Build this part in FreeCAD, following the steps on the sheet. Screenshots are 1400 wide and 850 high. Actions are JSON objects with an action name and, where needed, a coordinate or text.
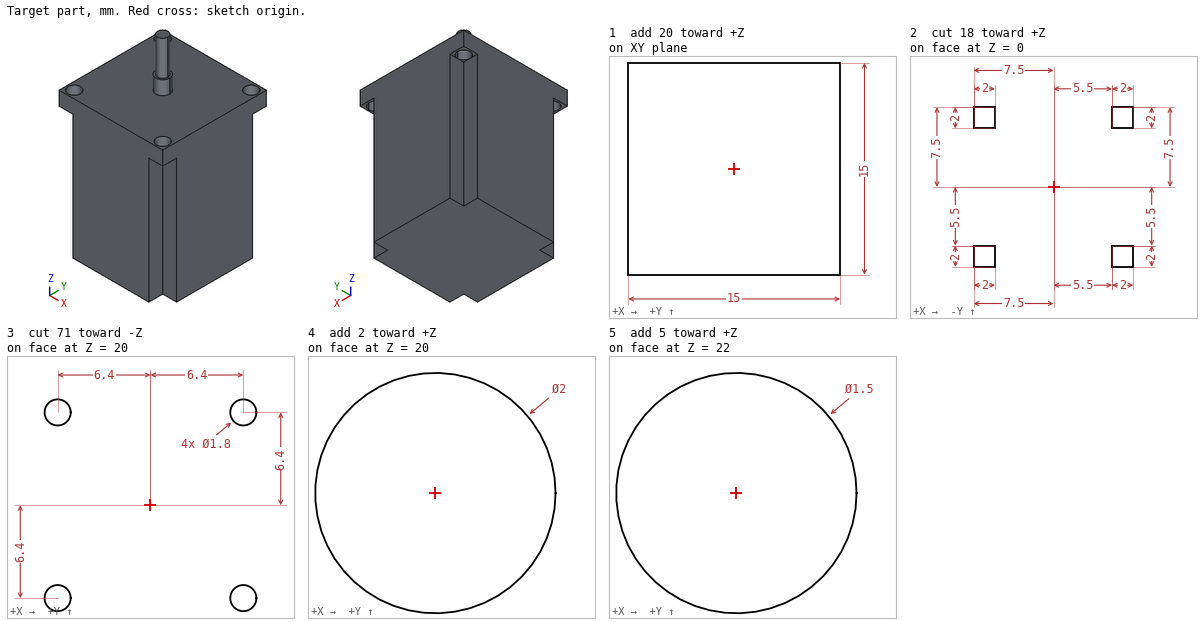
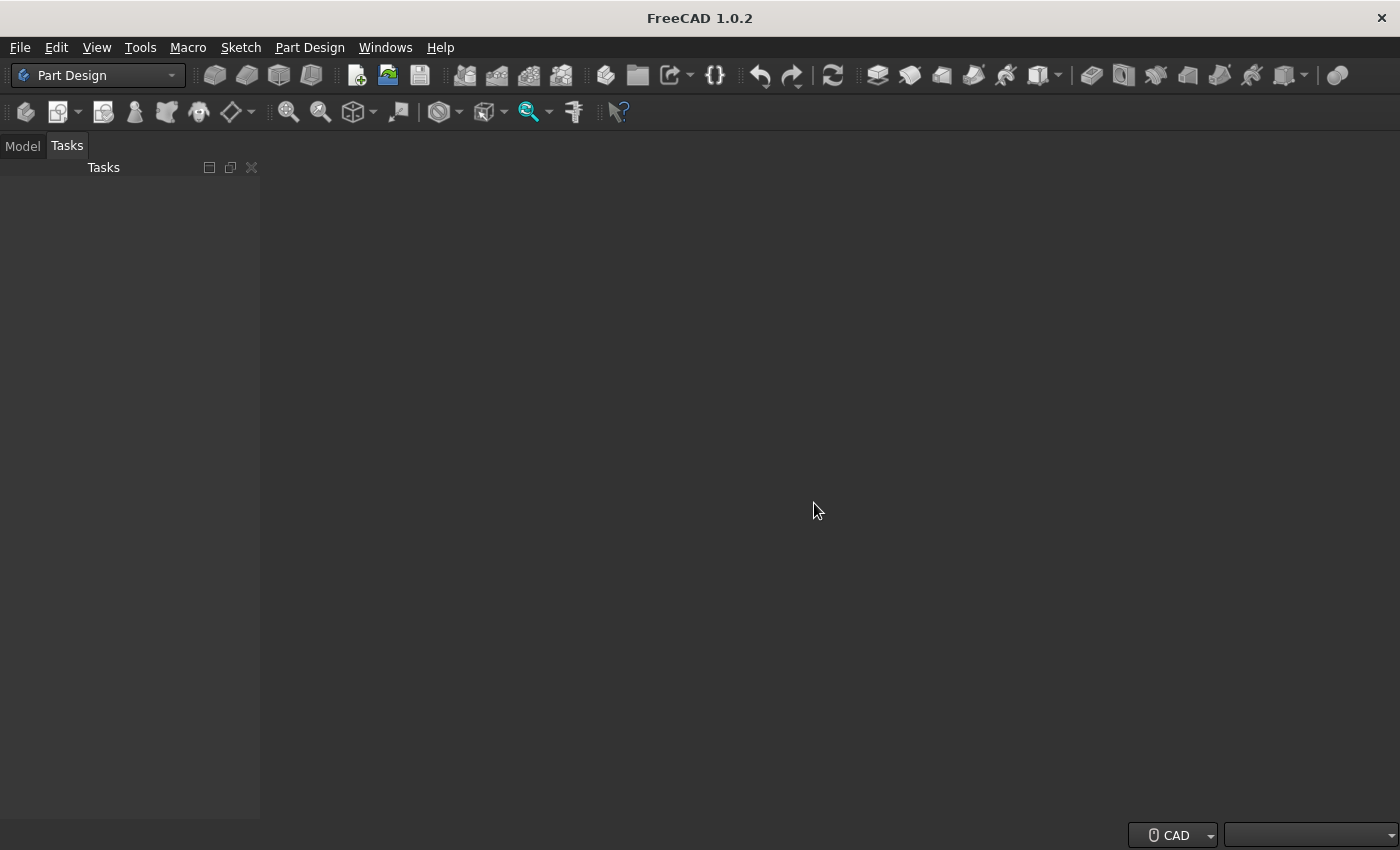
{"action": "left_click", "coordinate": [356, 76]}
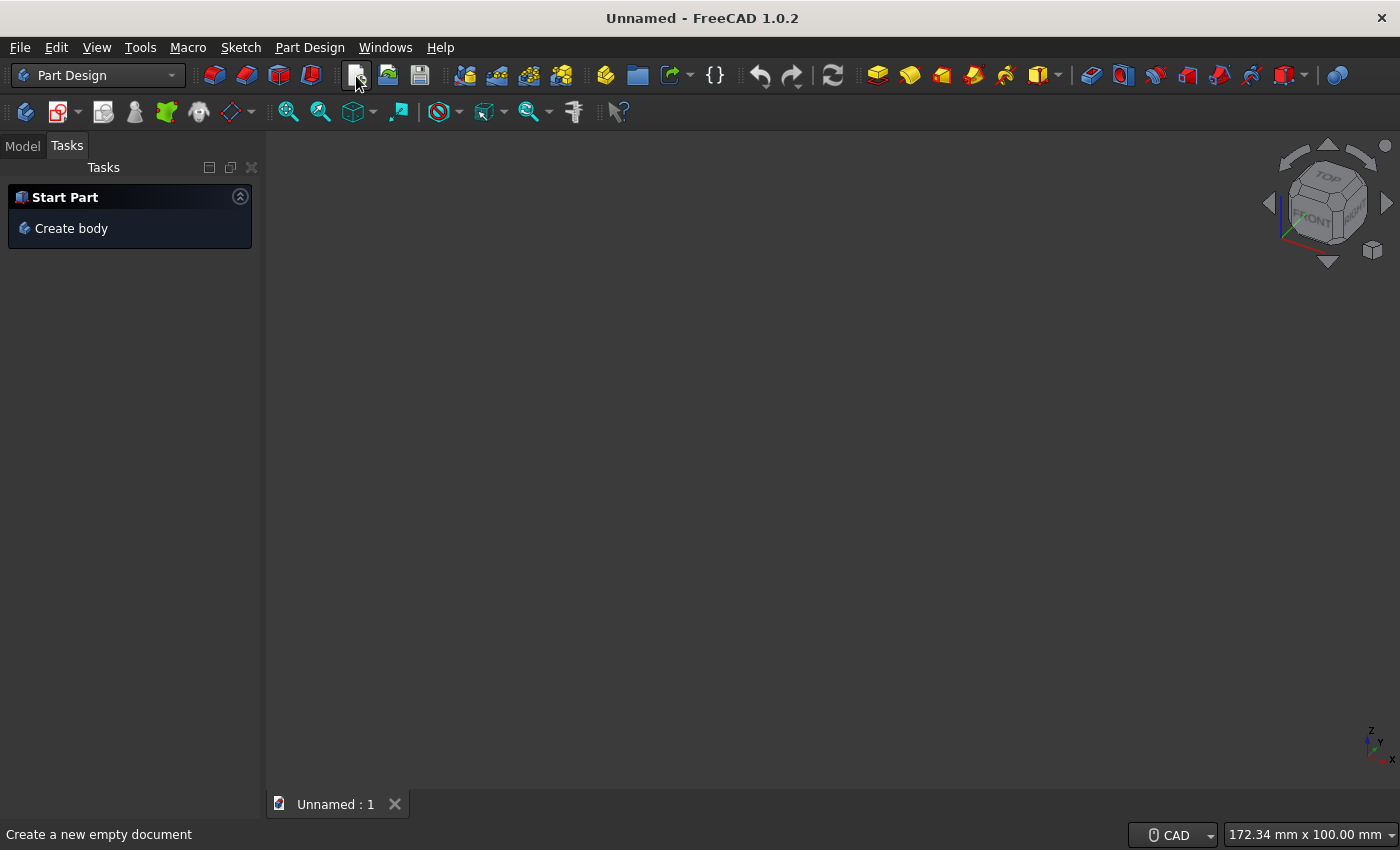
{"action": "left_click", "coordinate": [58, 112]}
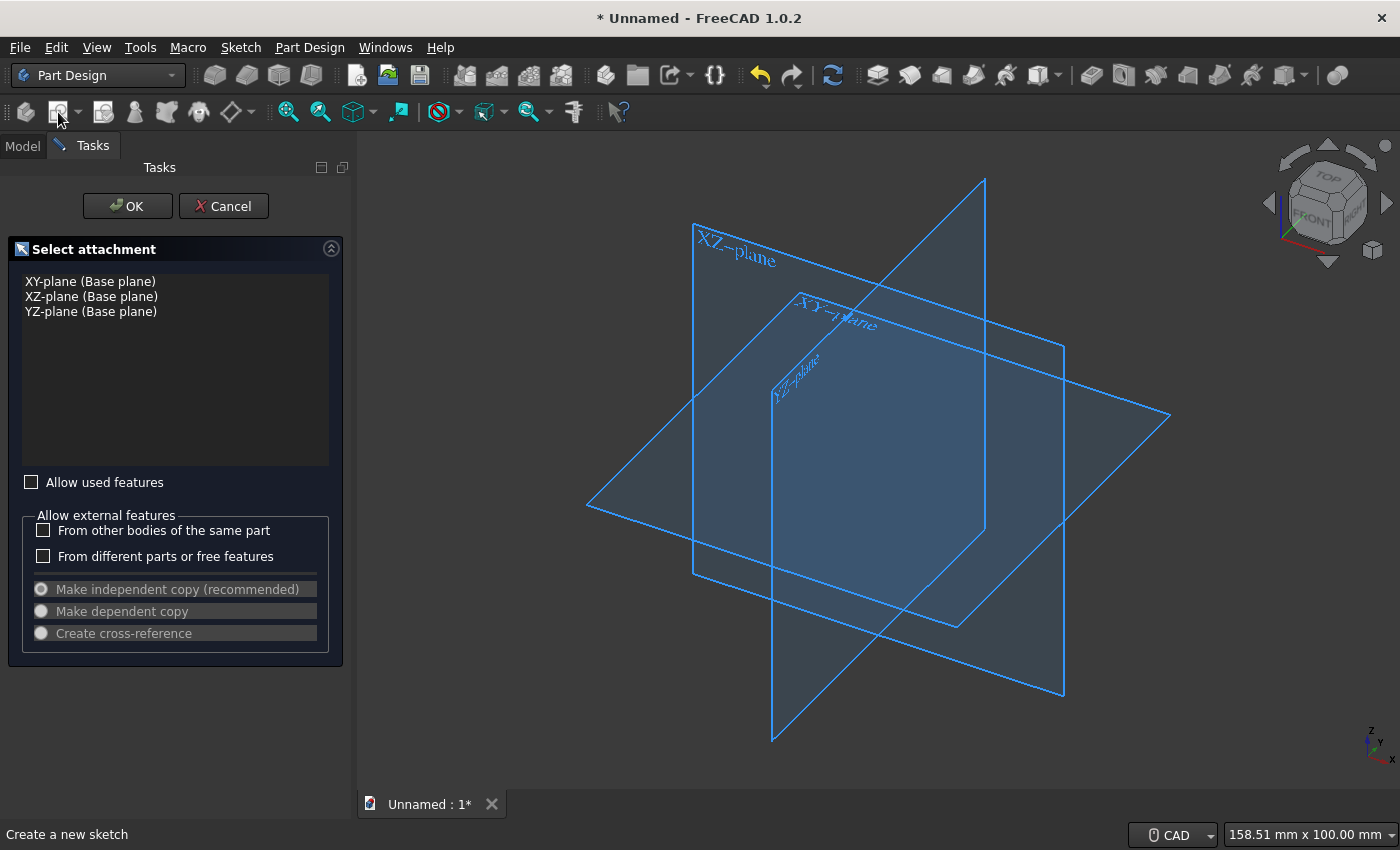
{"action": "left_click", "coordinate": [82, 282]}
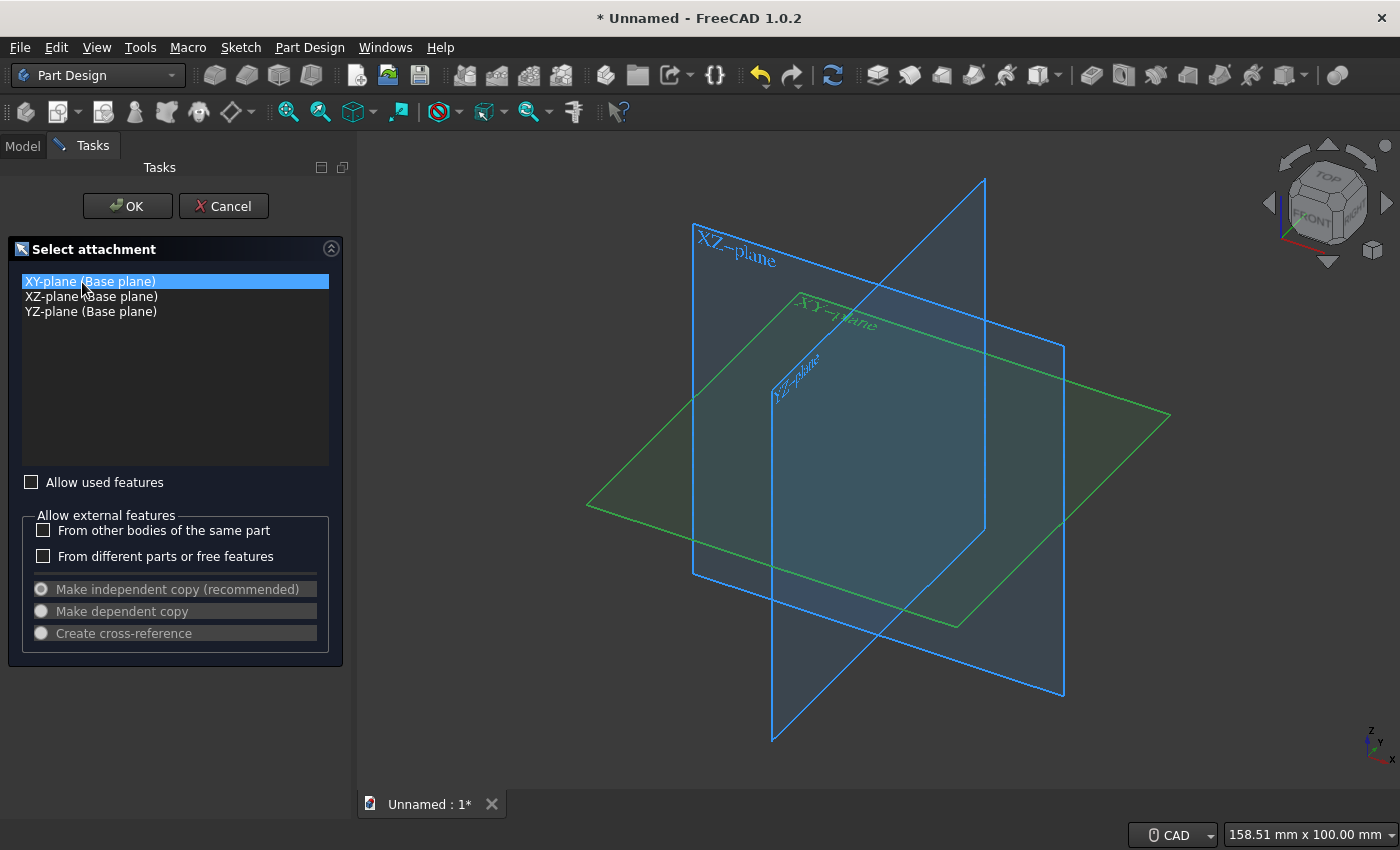
{"action": "left_click", "coordinate": [128, 206]}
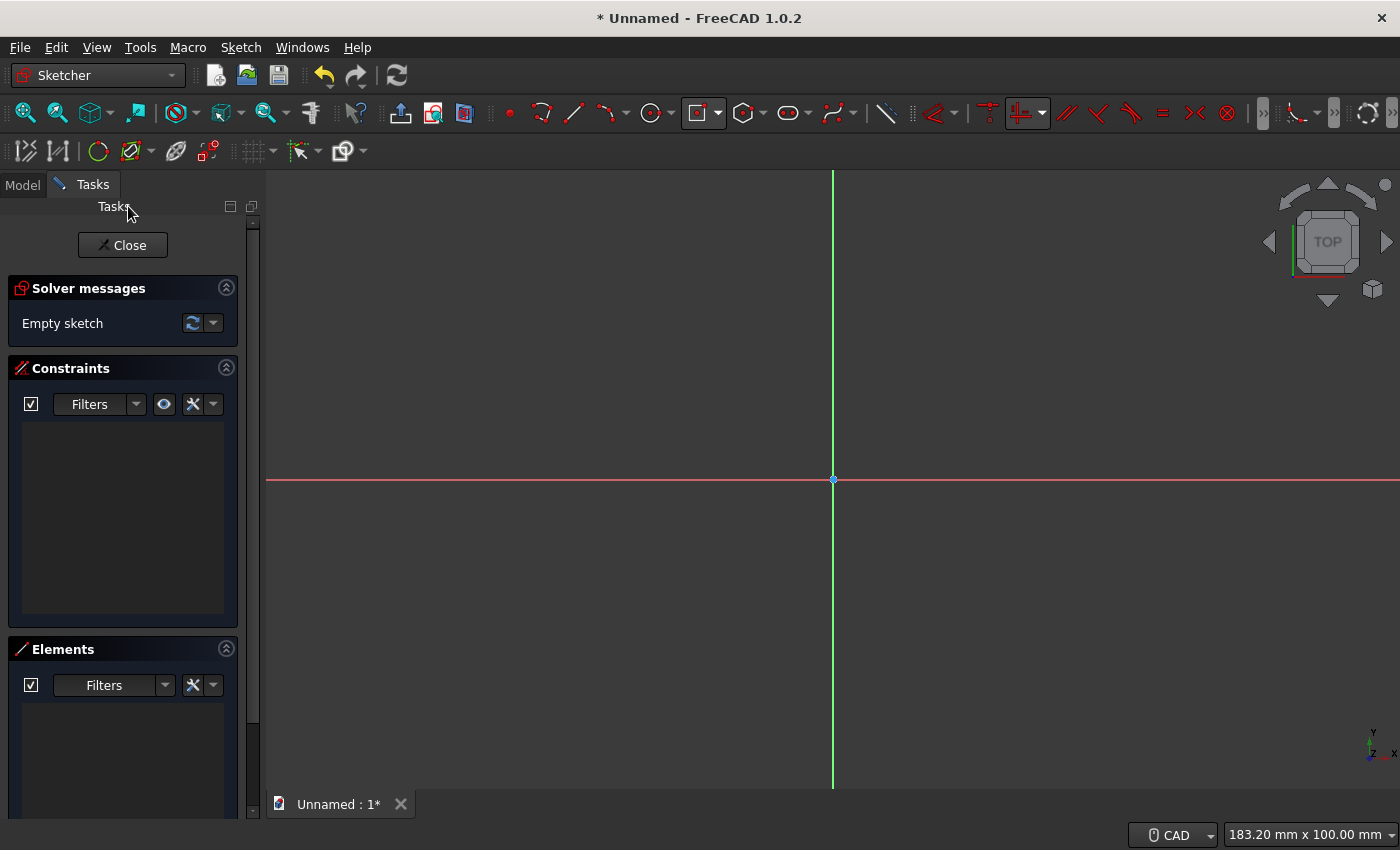
{"action": "scroll", "coordinate": [855, 480], "scroll_direction": "up", "scroll_amount": 7}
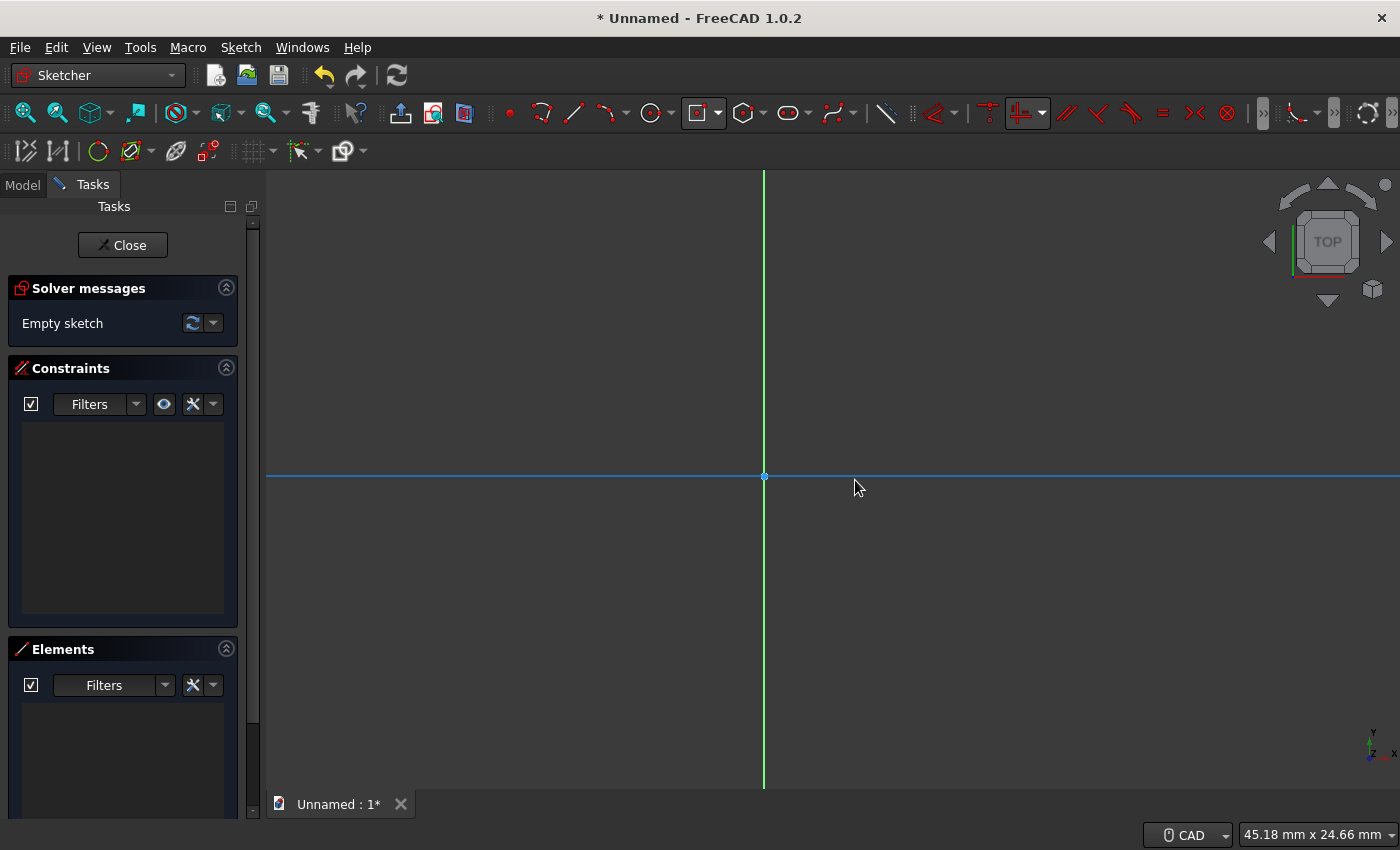
{"action": "key", "text": "g v"}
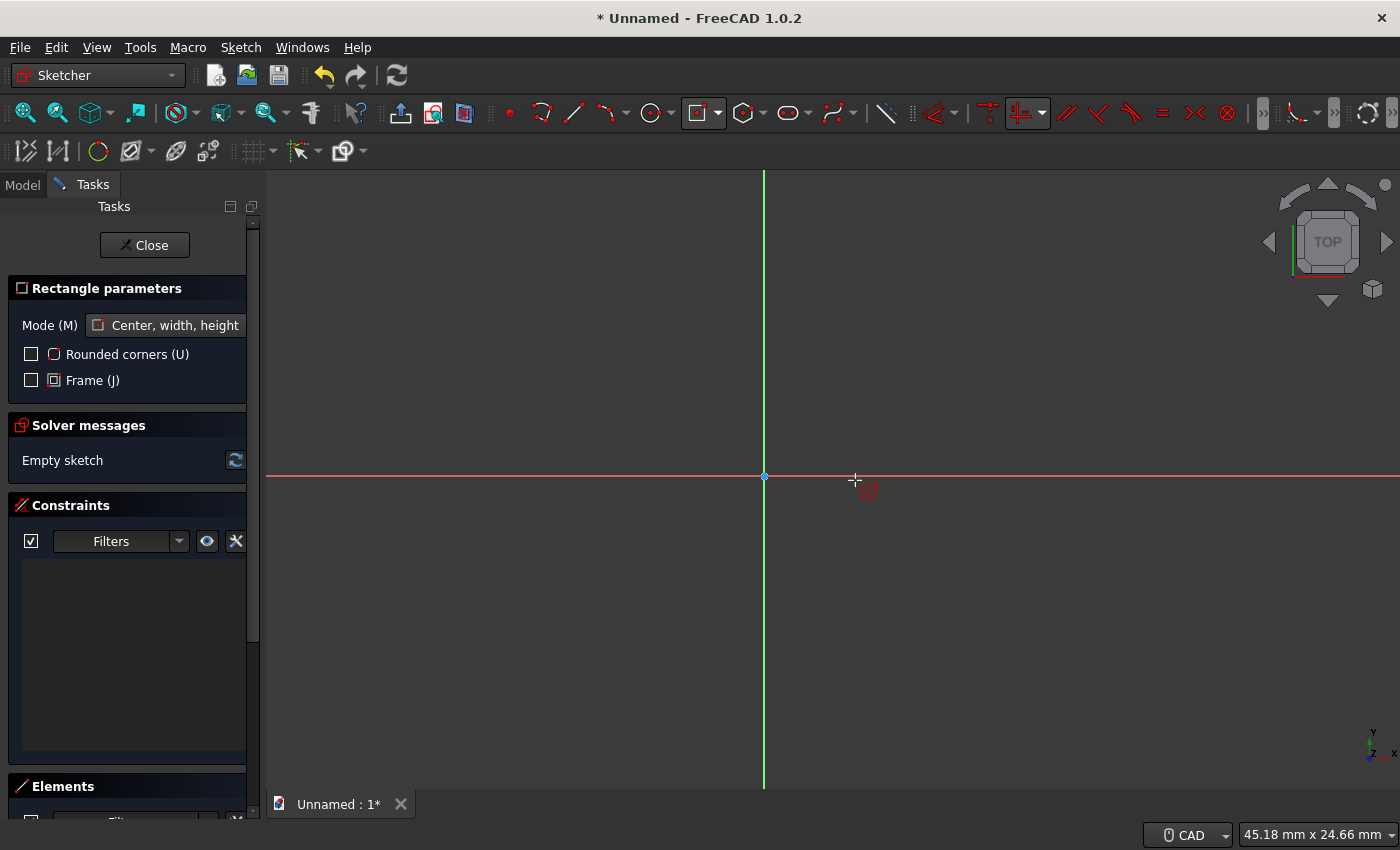
{"action": "left_click", "coordinate": [764, 476]}
{"action": "mouse_move", "coordinate": [952, 288]}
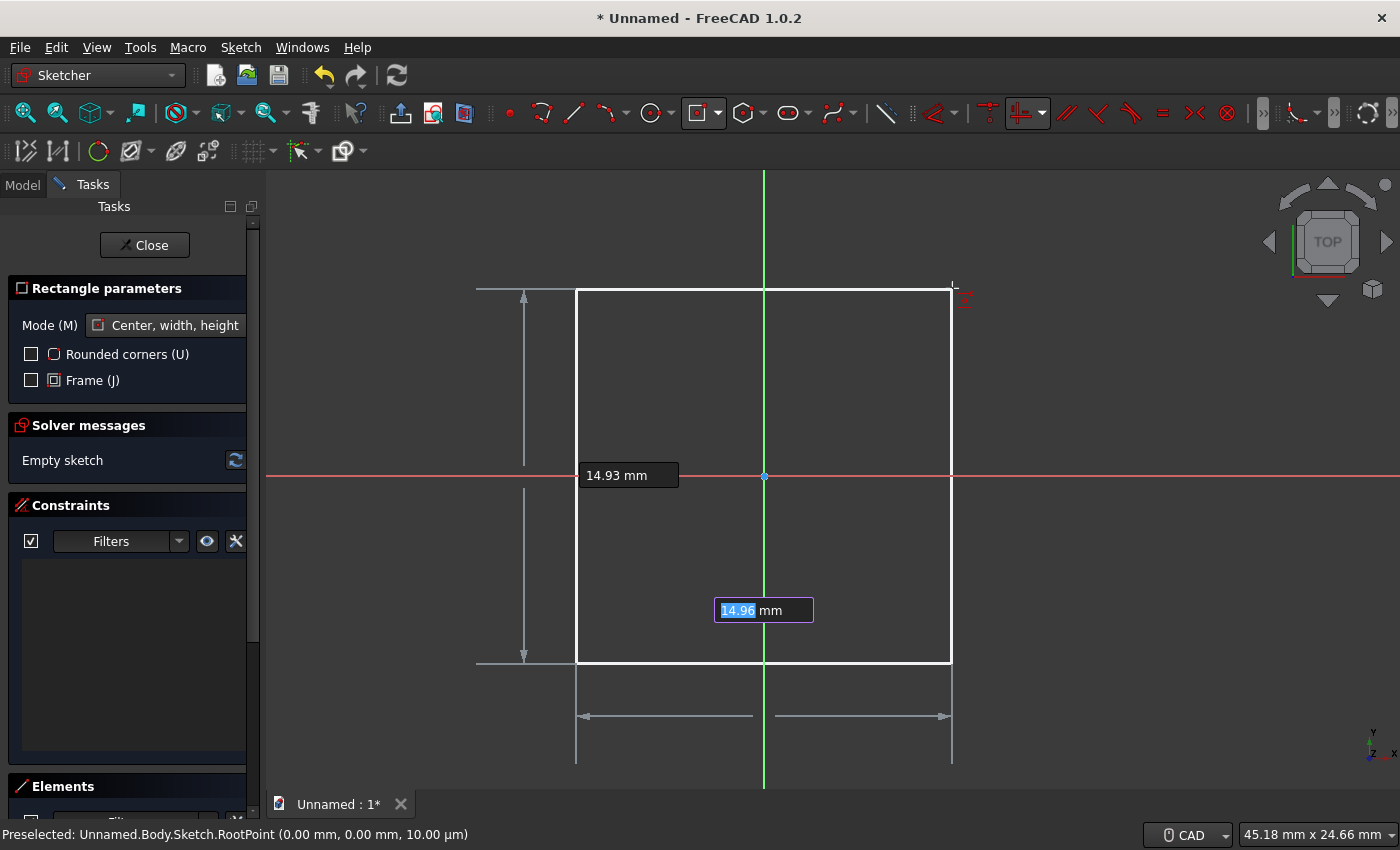
{"action": "type", "text": "15"}
{"action": "key", "text": "Tab"}
{"action": "type", "text": "15"}
{"action": "key", "text": "Return"}
{"action": "key", "text": "Escape"}